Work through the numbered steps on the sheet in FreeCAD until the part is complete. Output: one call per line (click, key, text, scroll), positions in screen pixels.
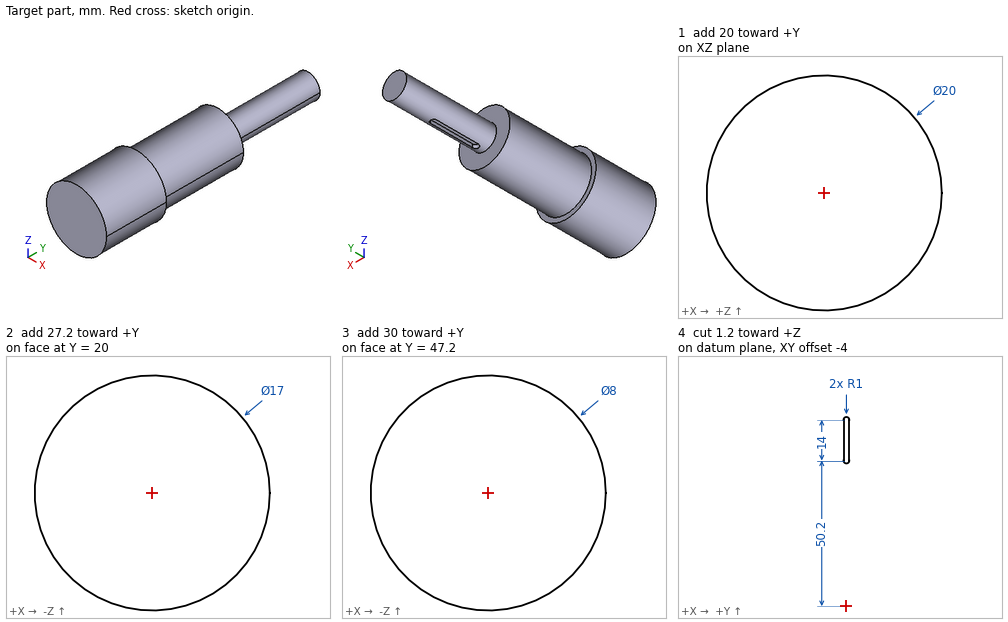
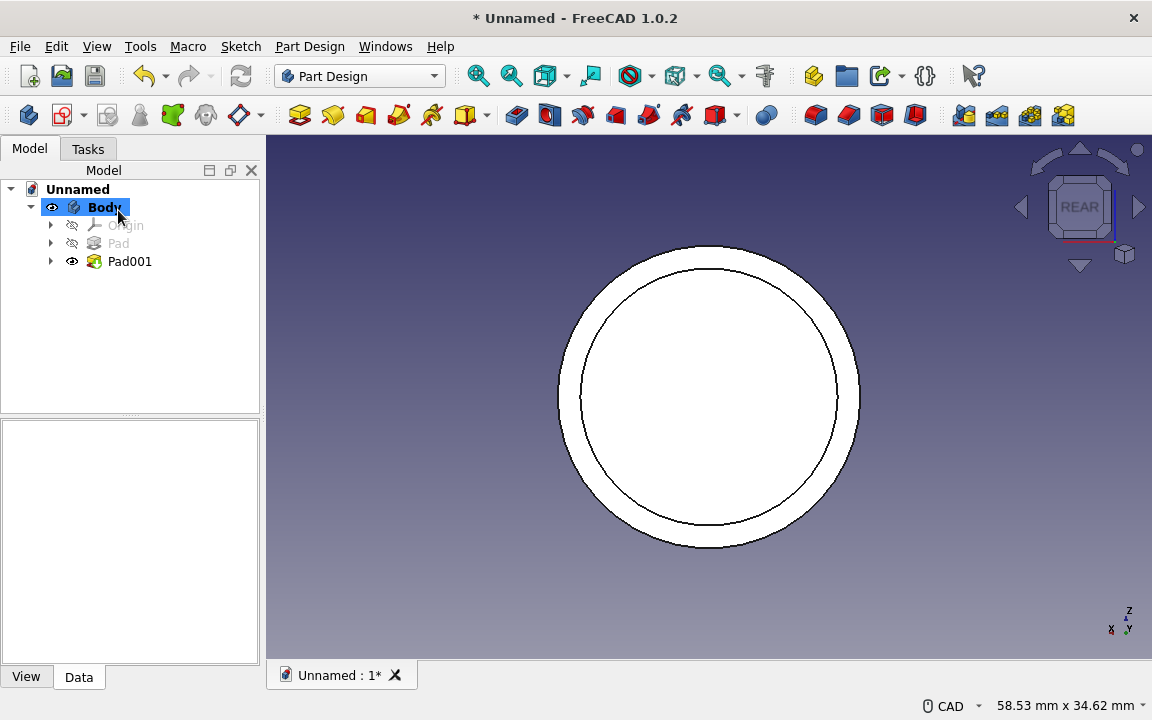
click(709, 396)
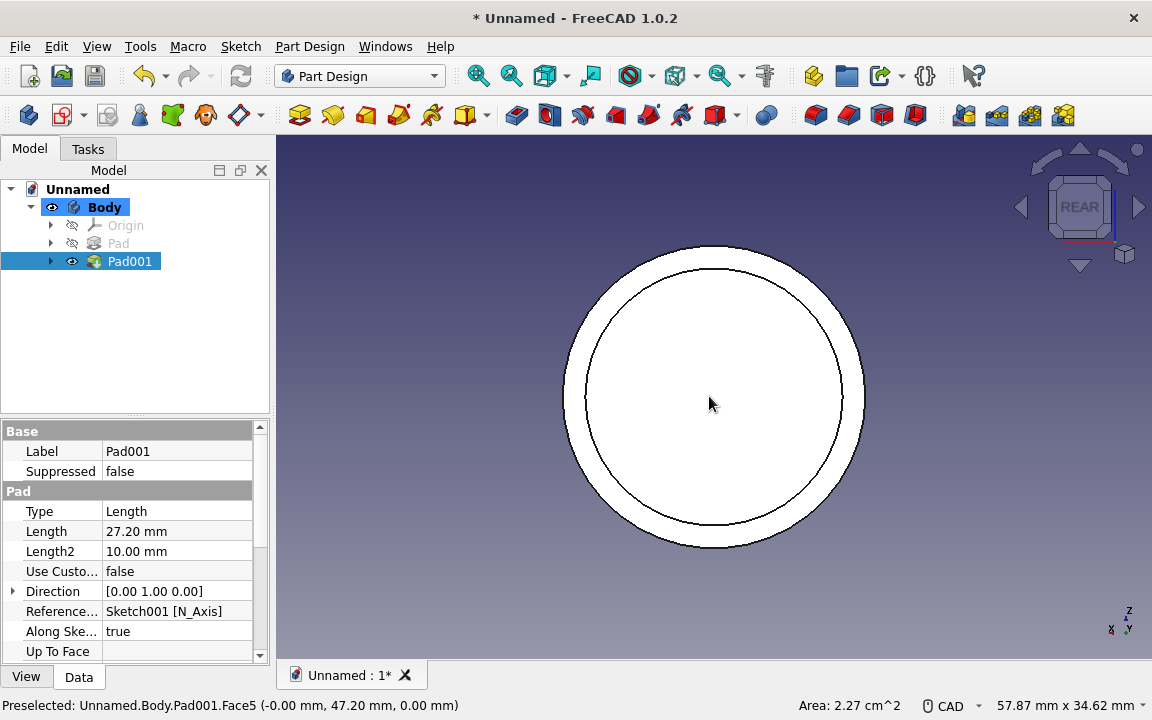
click(62, 116)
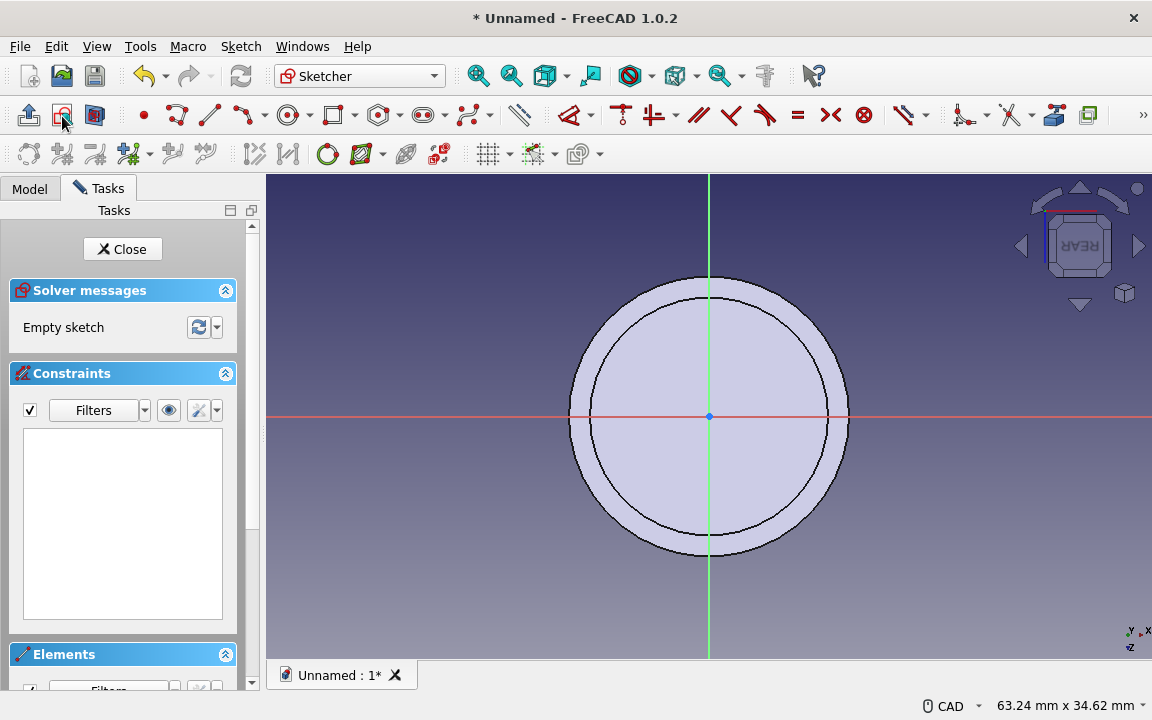
scroll(749, 416, up, 5)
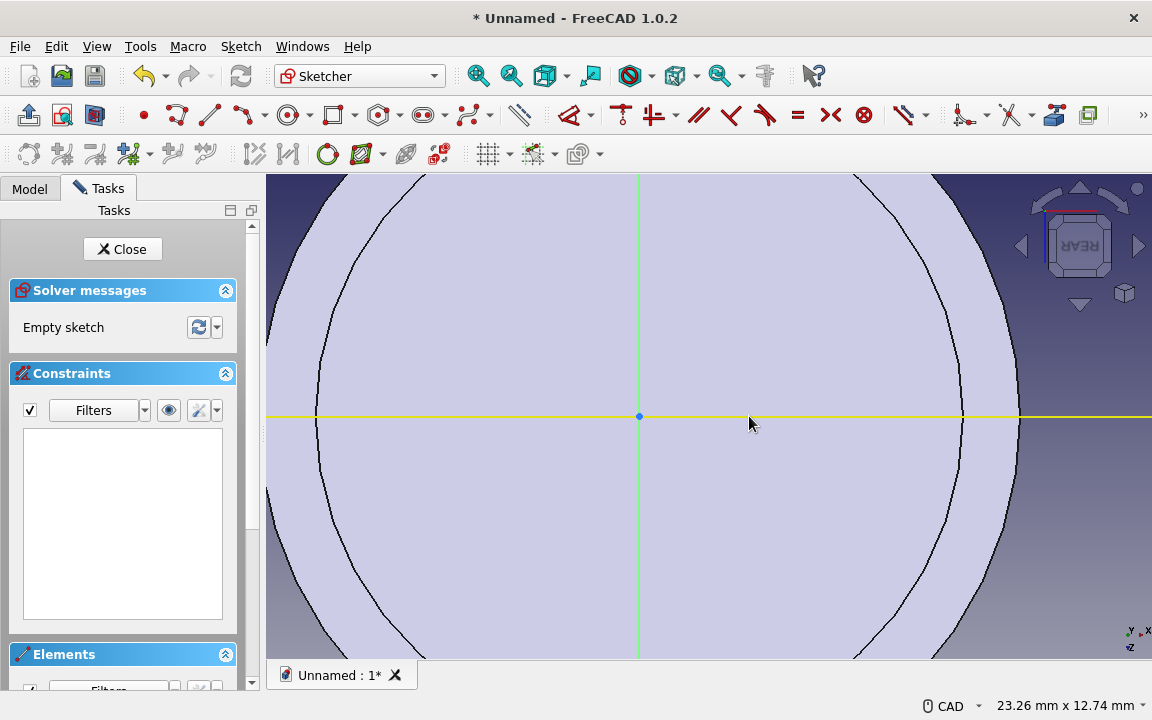
click(288, 116)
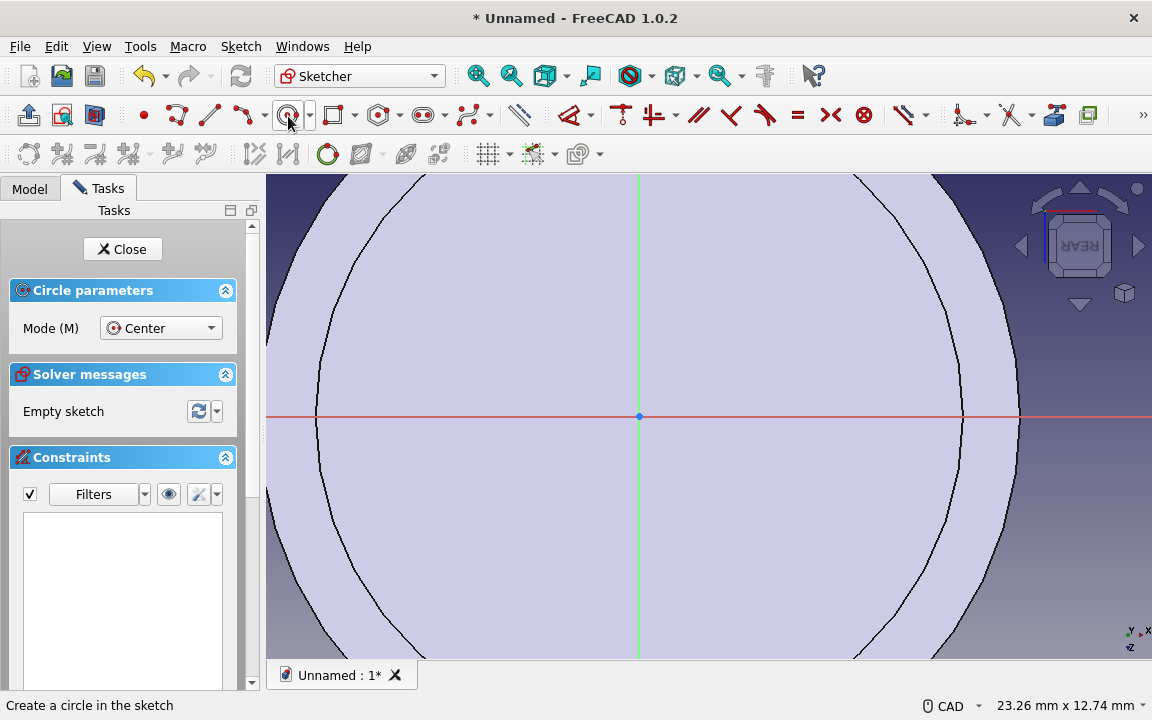
click(639, 416)
move(747, 309)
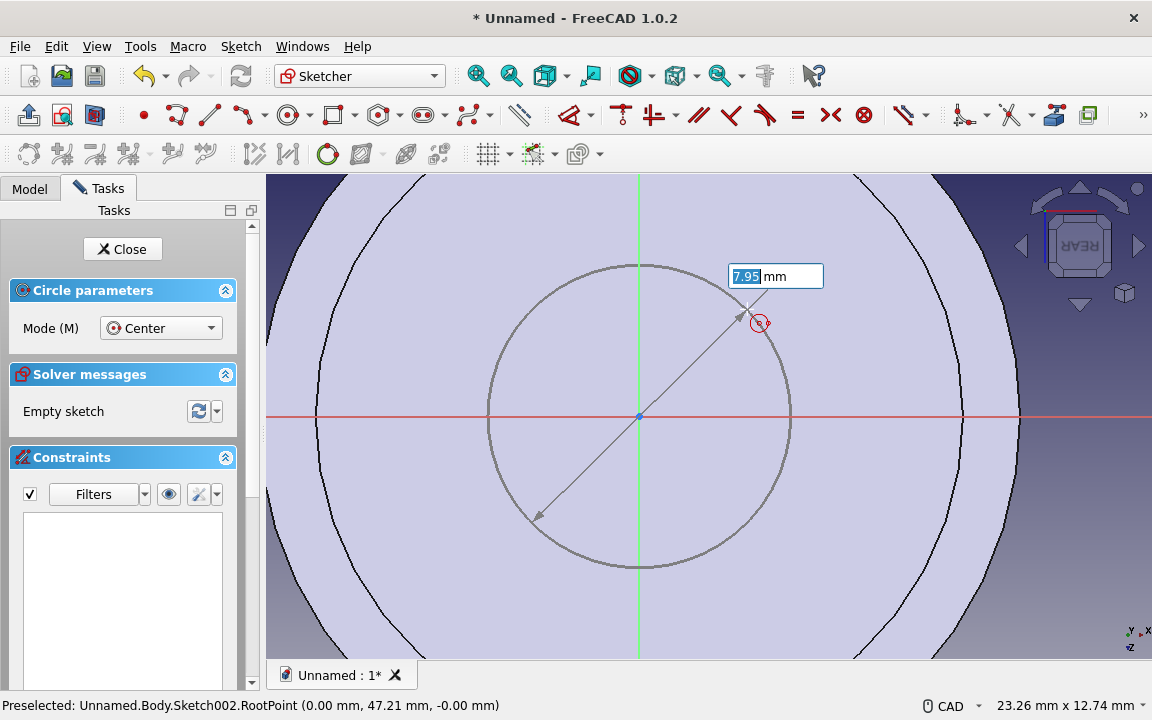
text(8)
key(Return)
key(Escape)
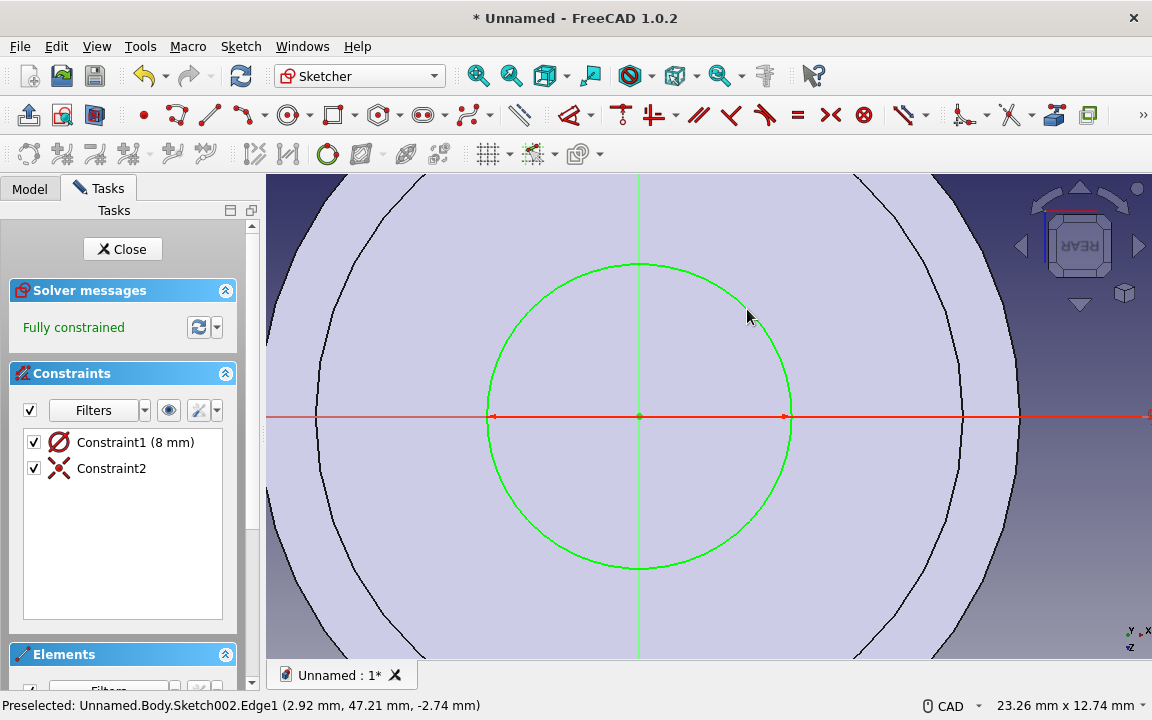
click(123, 249)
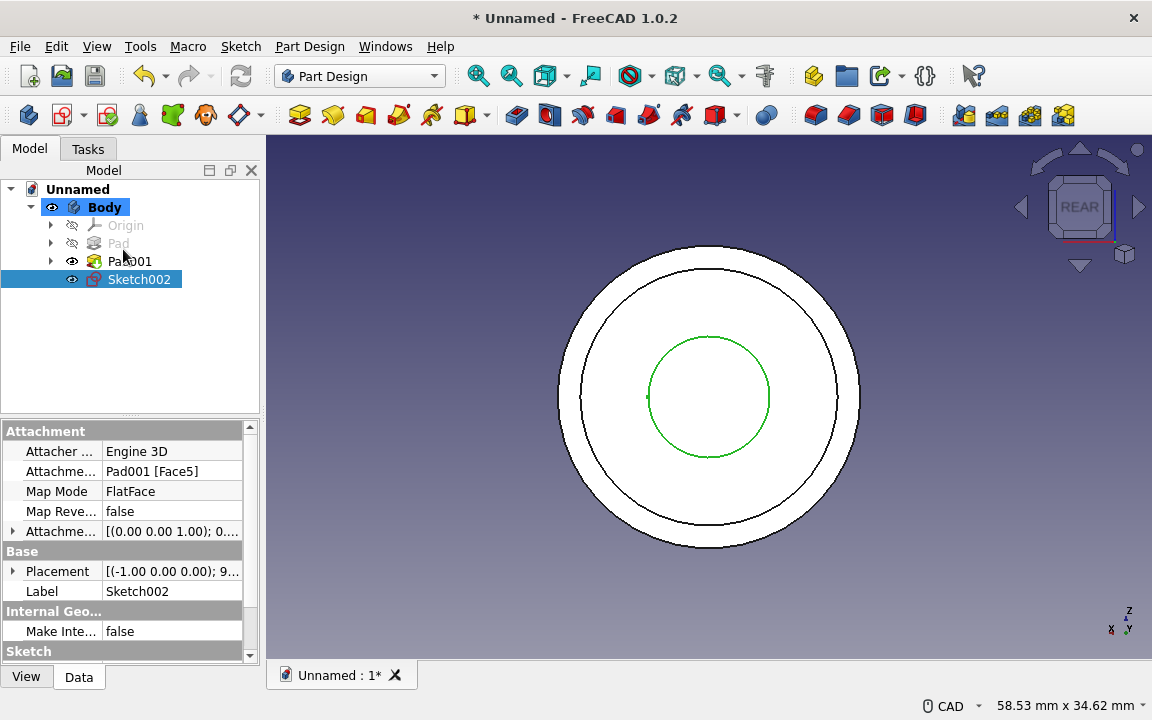
click(300, 116)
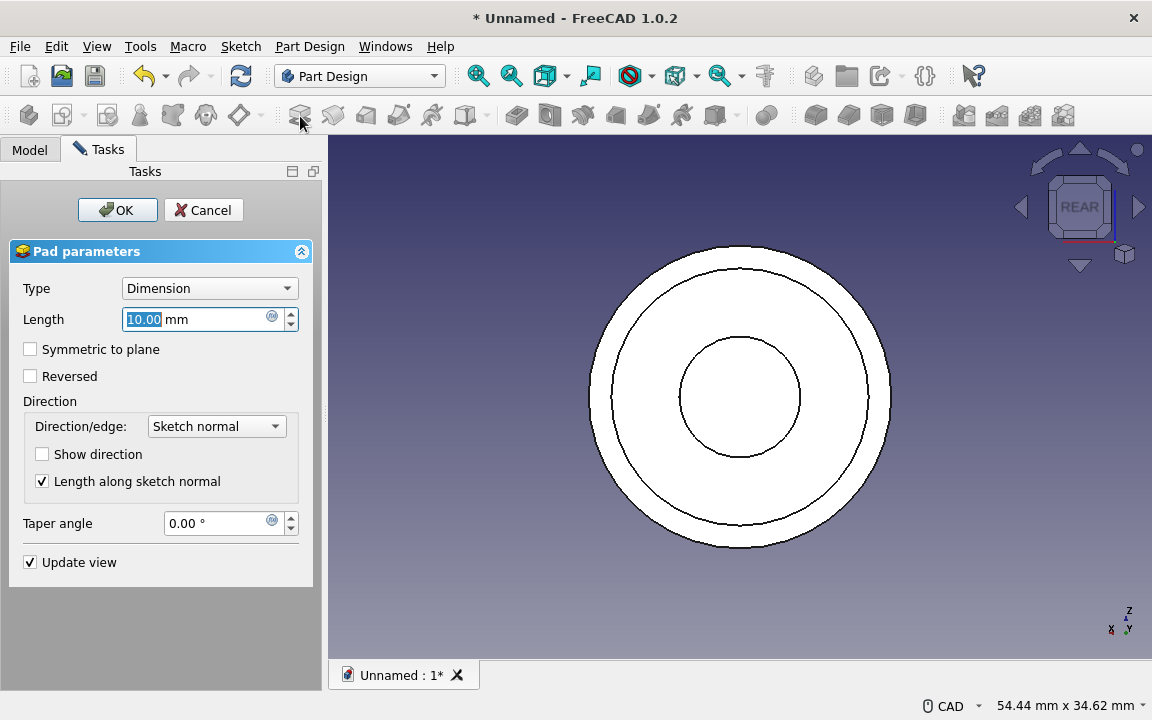
text(30)
key(Tab)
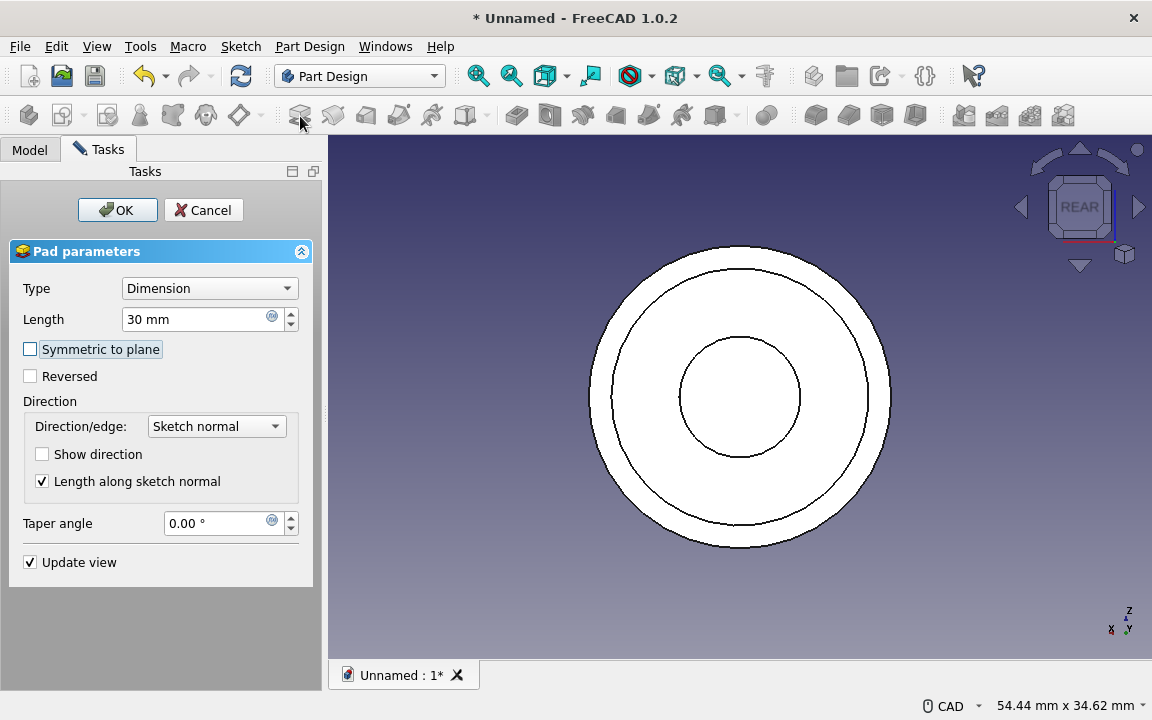
click(118, 210)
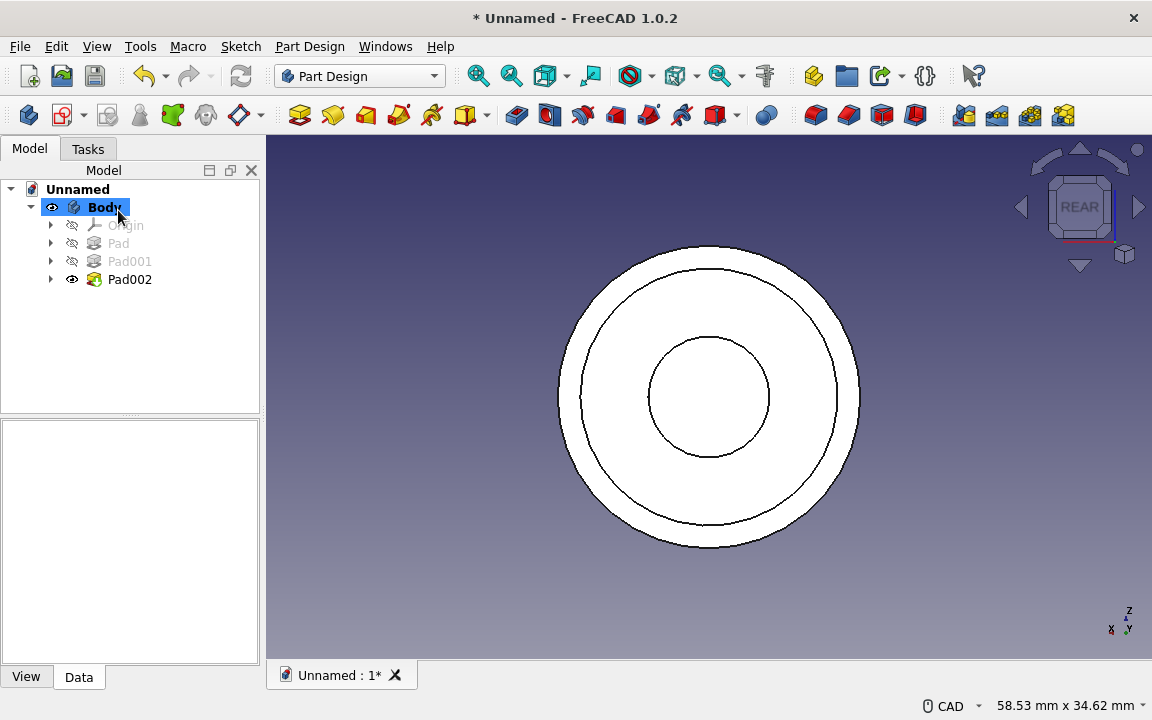
click(51, 225)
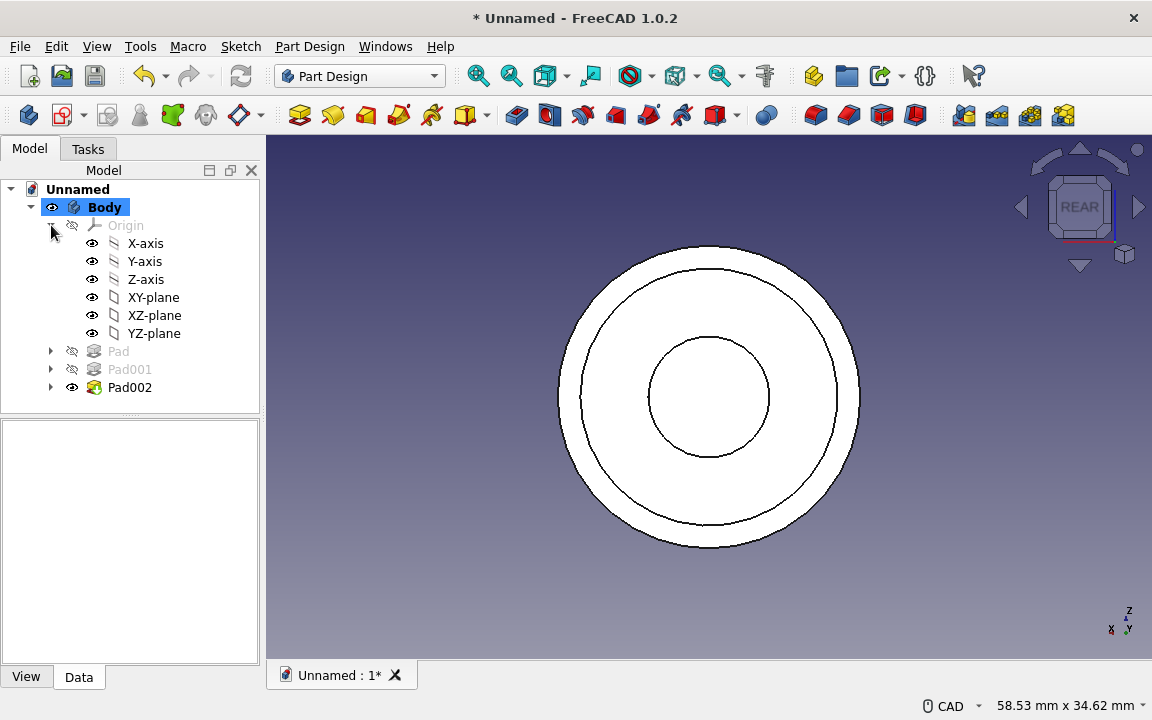
click(137, 297)